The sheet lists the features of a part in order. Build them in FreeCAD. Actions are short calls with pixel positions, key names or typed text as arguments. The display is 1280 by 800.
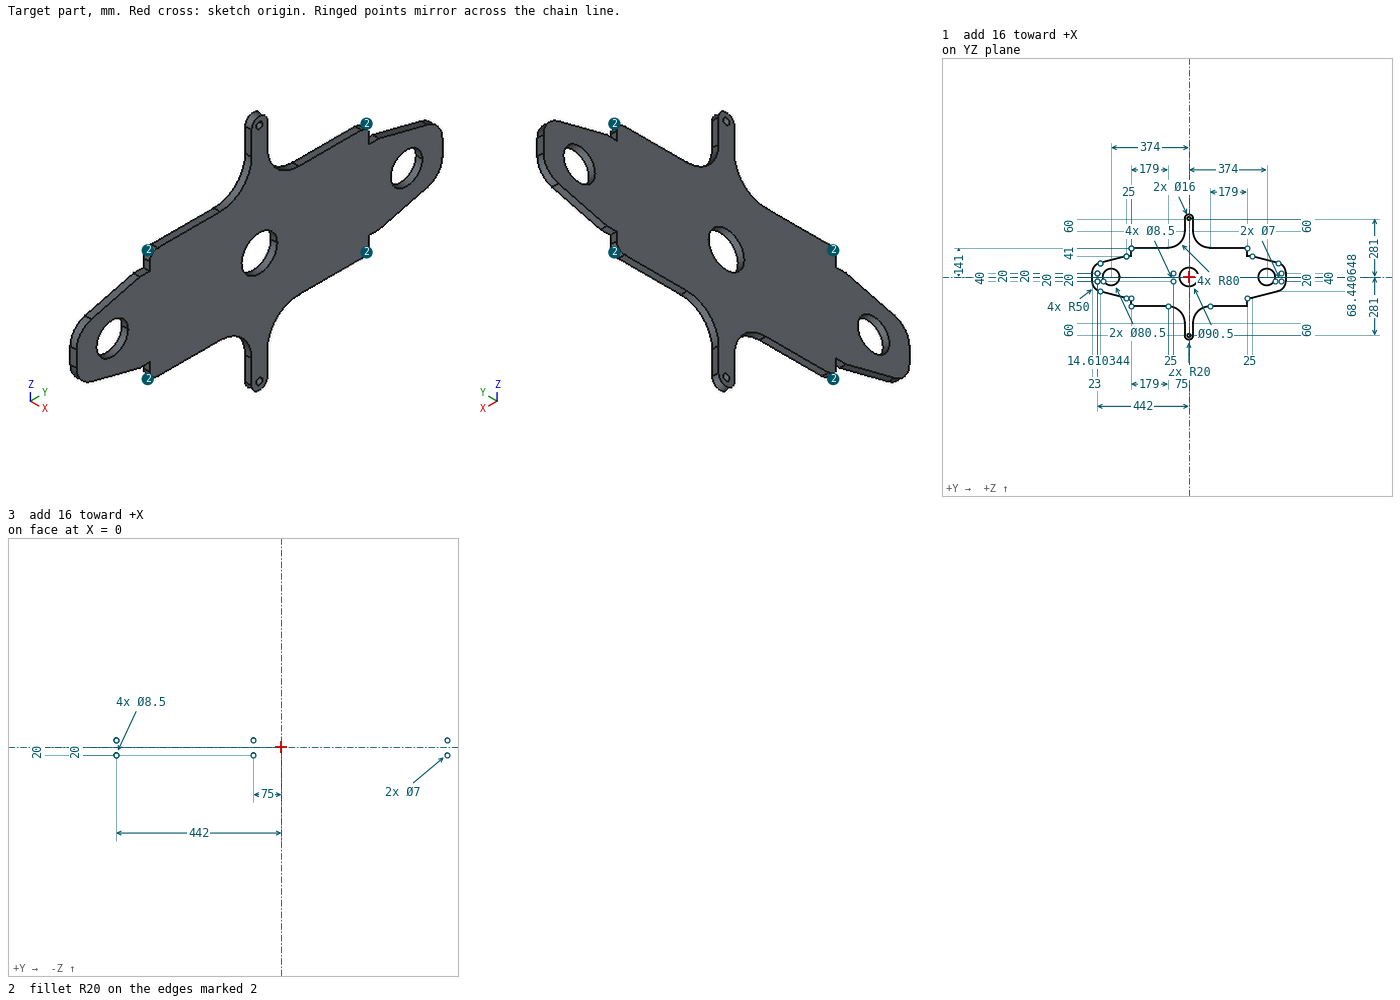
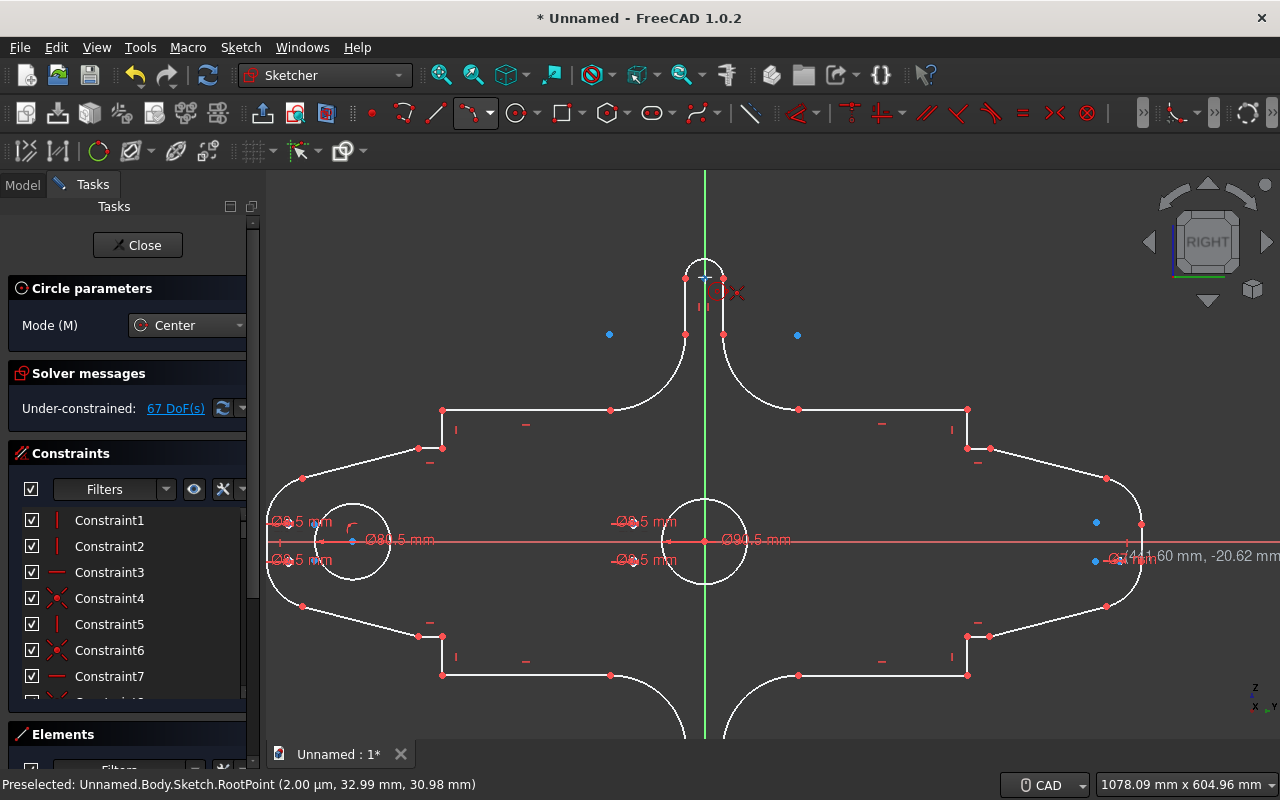
click(705, 277)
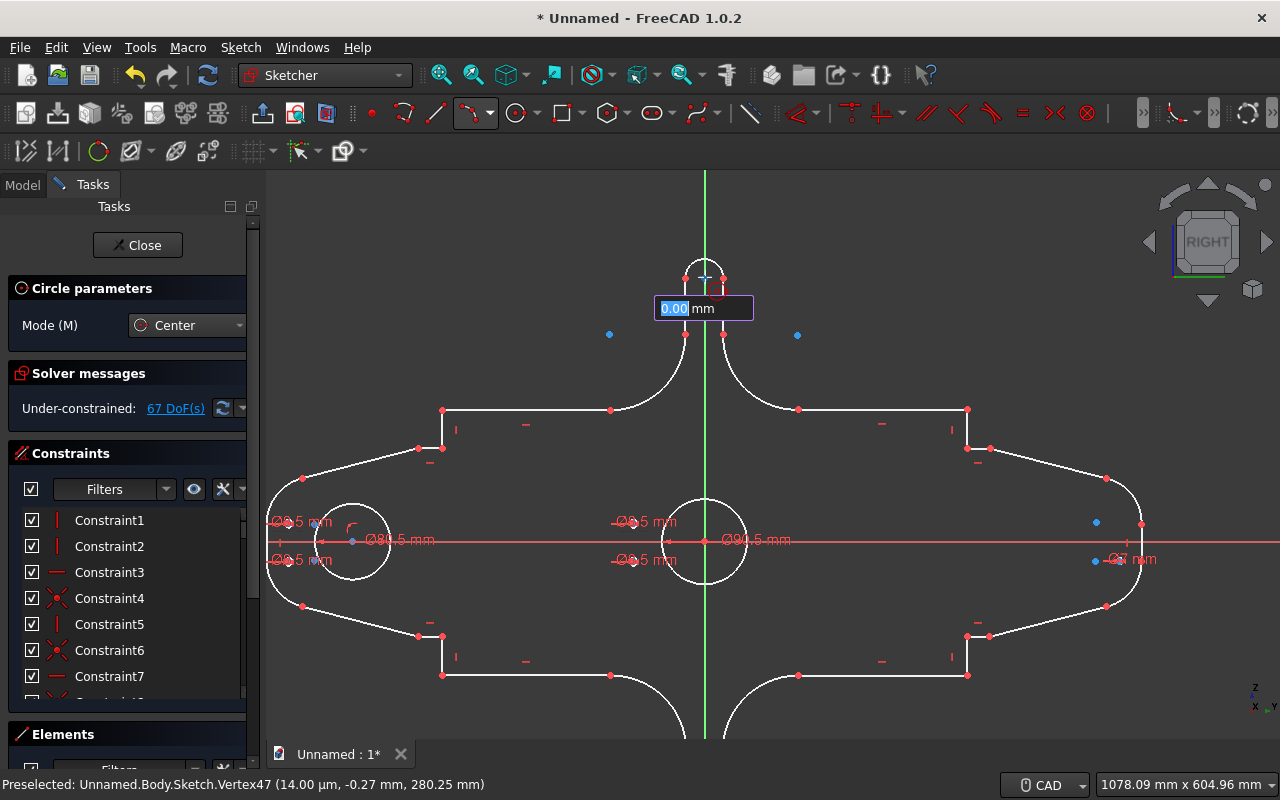
scroll(712, 275, up, 5)
move(710, 274)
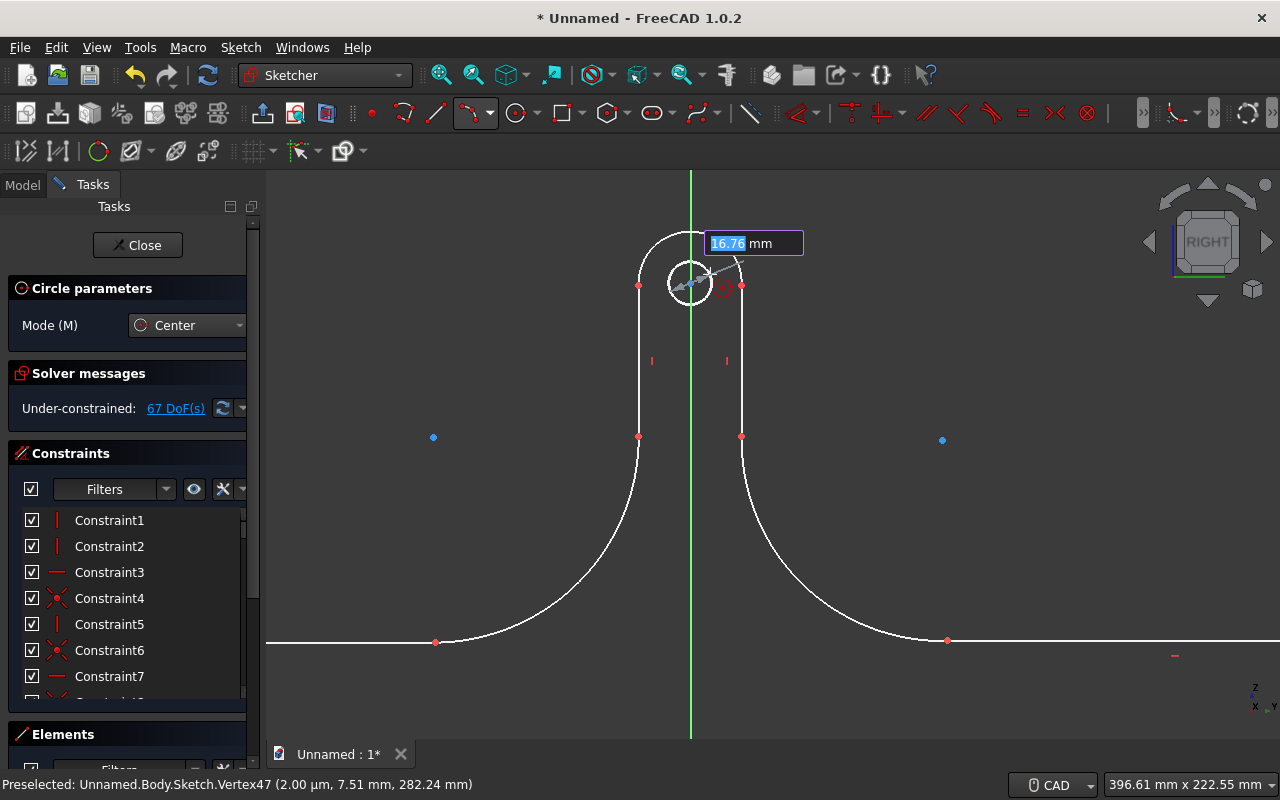
text(16)
key(Return)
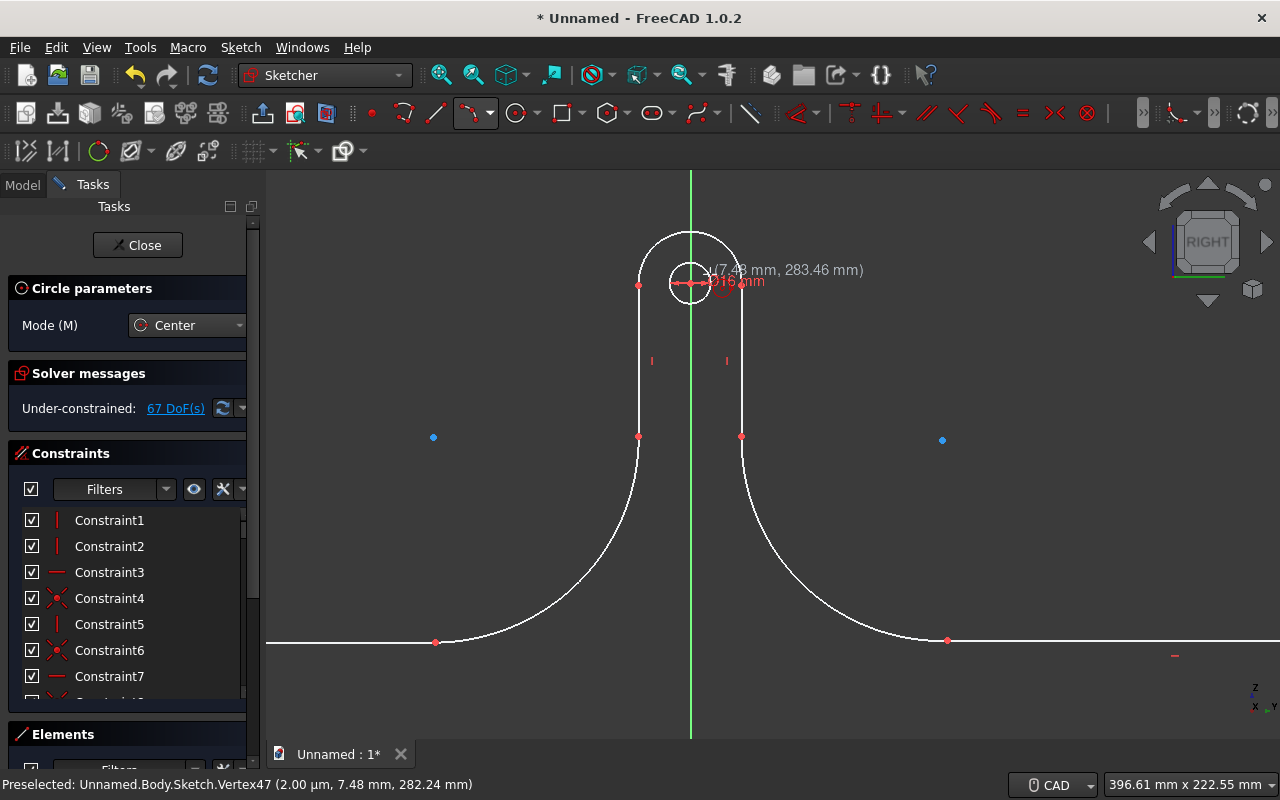
scroll(709, 276, down, 7)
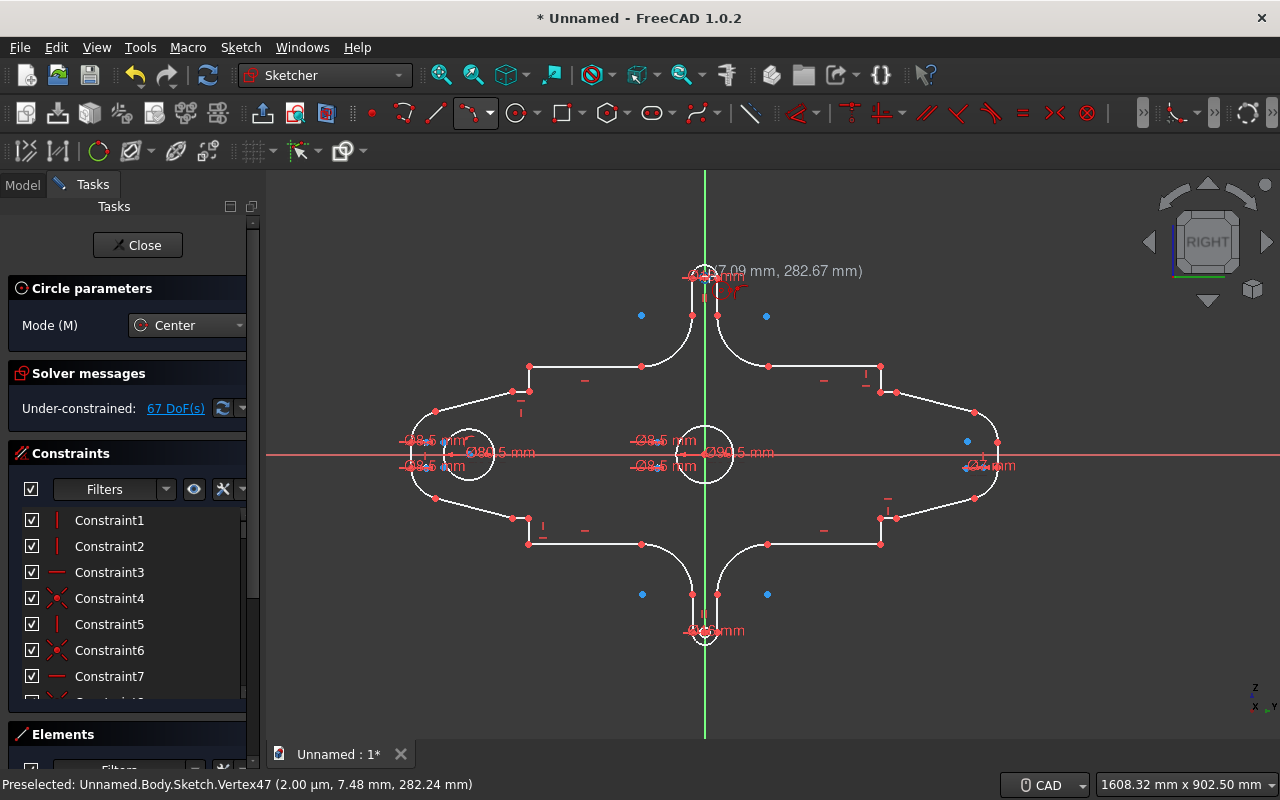
click(941, 455)
move(923, 437)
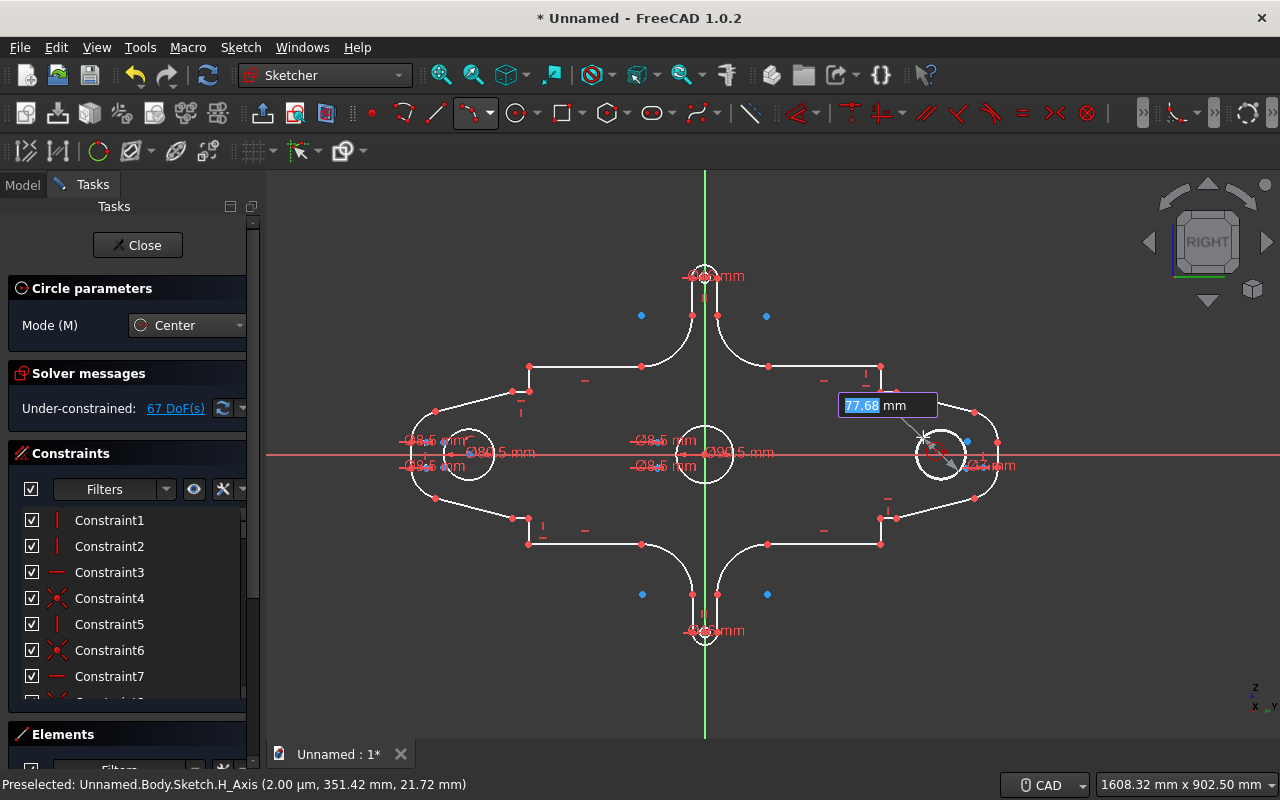
text(80.5)
key(Return)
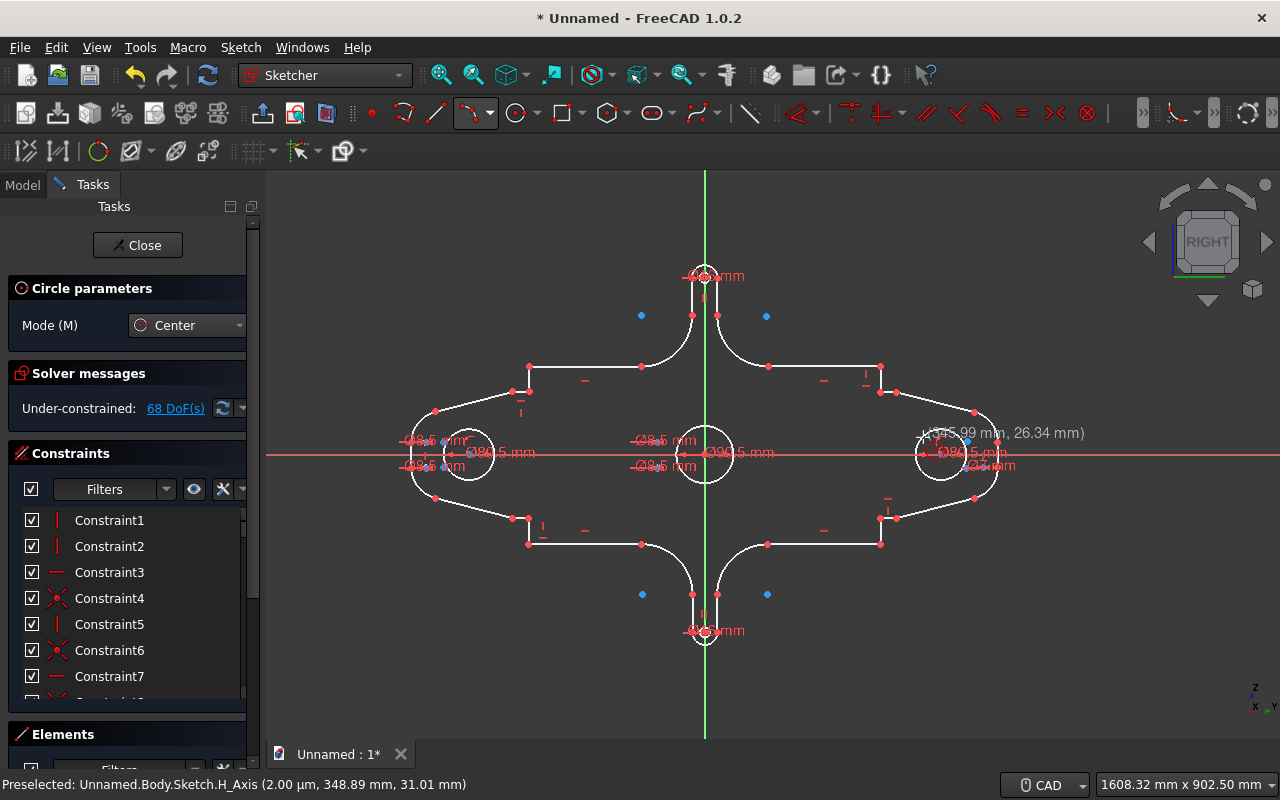
scroll(984, 442, up, 12)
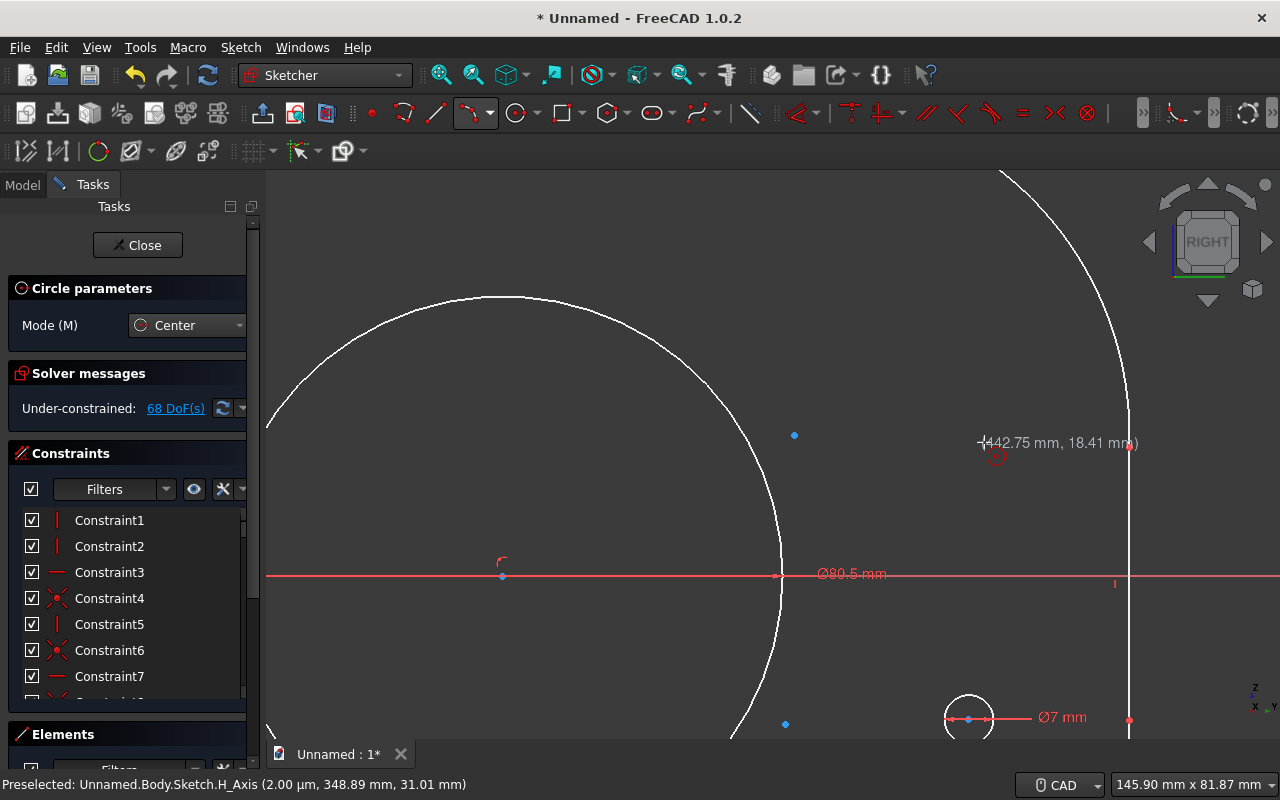
scroll(984, 442, down, 12)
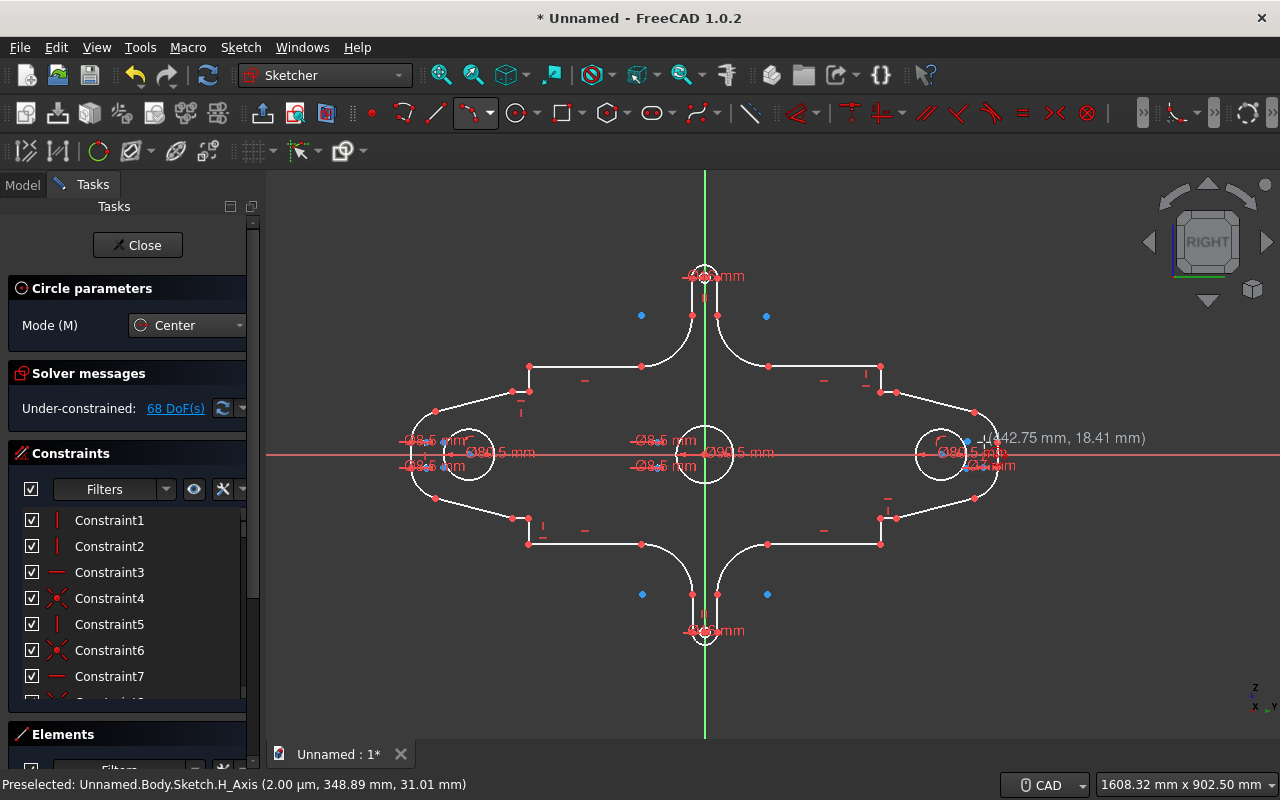
scroll(984, 442, up, 2)